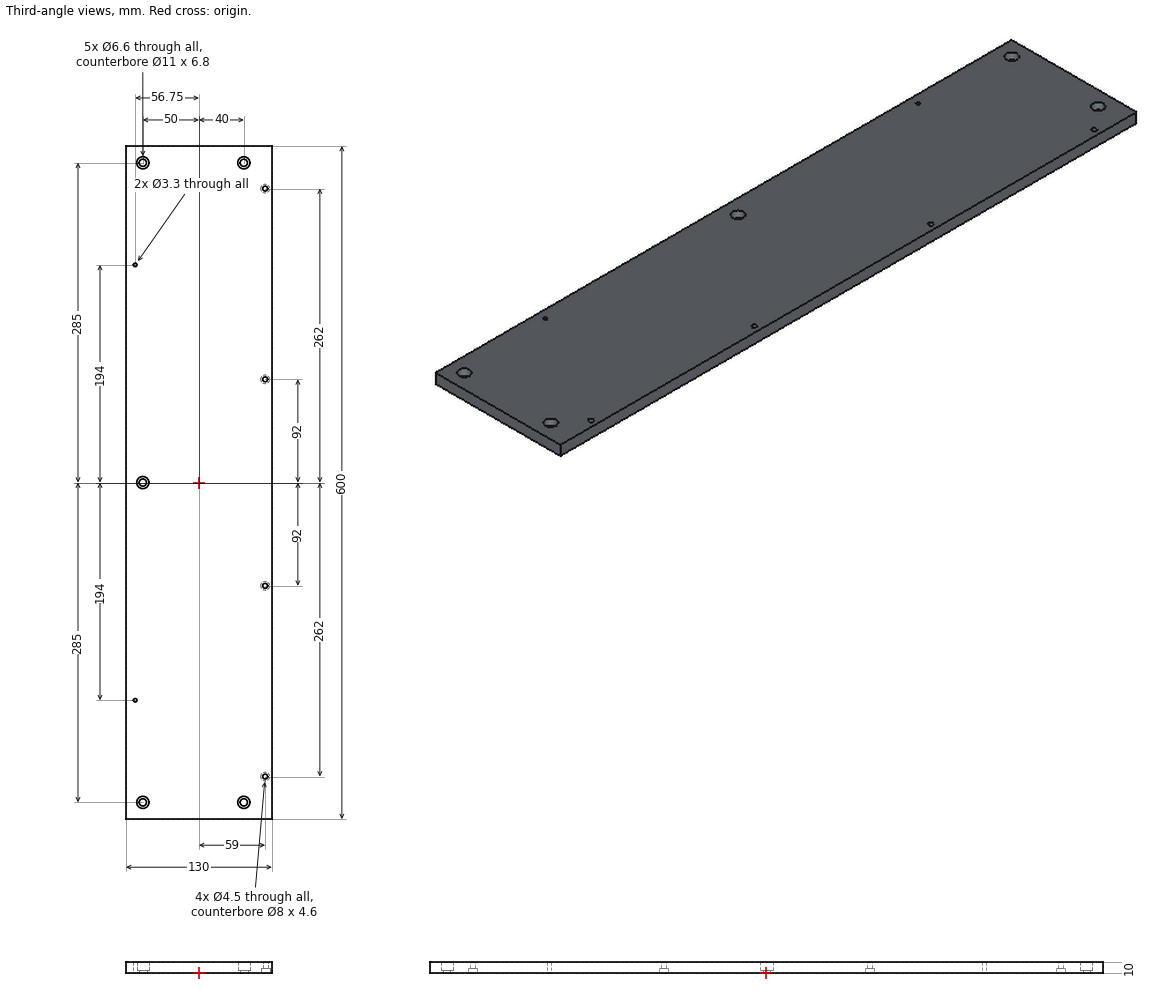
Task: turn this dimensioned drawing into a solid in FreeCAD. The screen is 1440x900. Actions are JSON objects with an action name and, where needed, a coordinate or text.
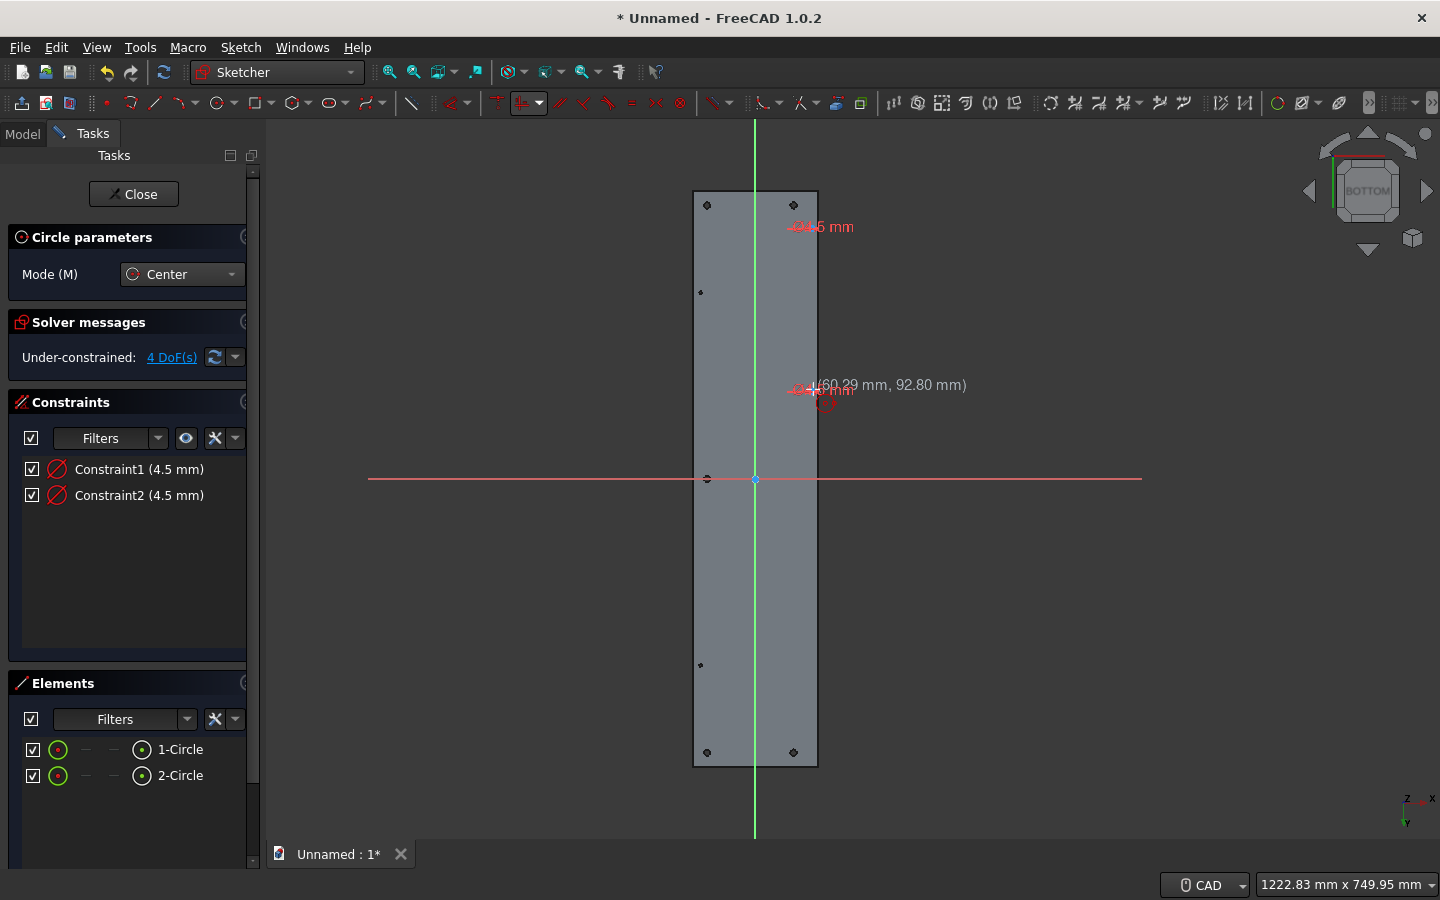
{"action": "scroll", "coordinate": [812, 567], "scroll_direction": "up", "scroll_amount": 12}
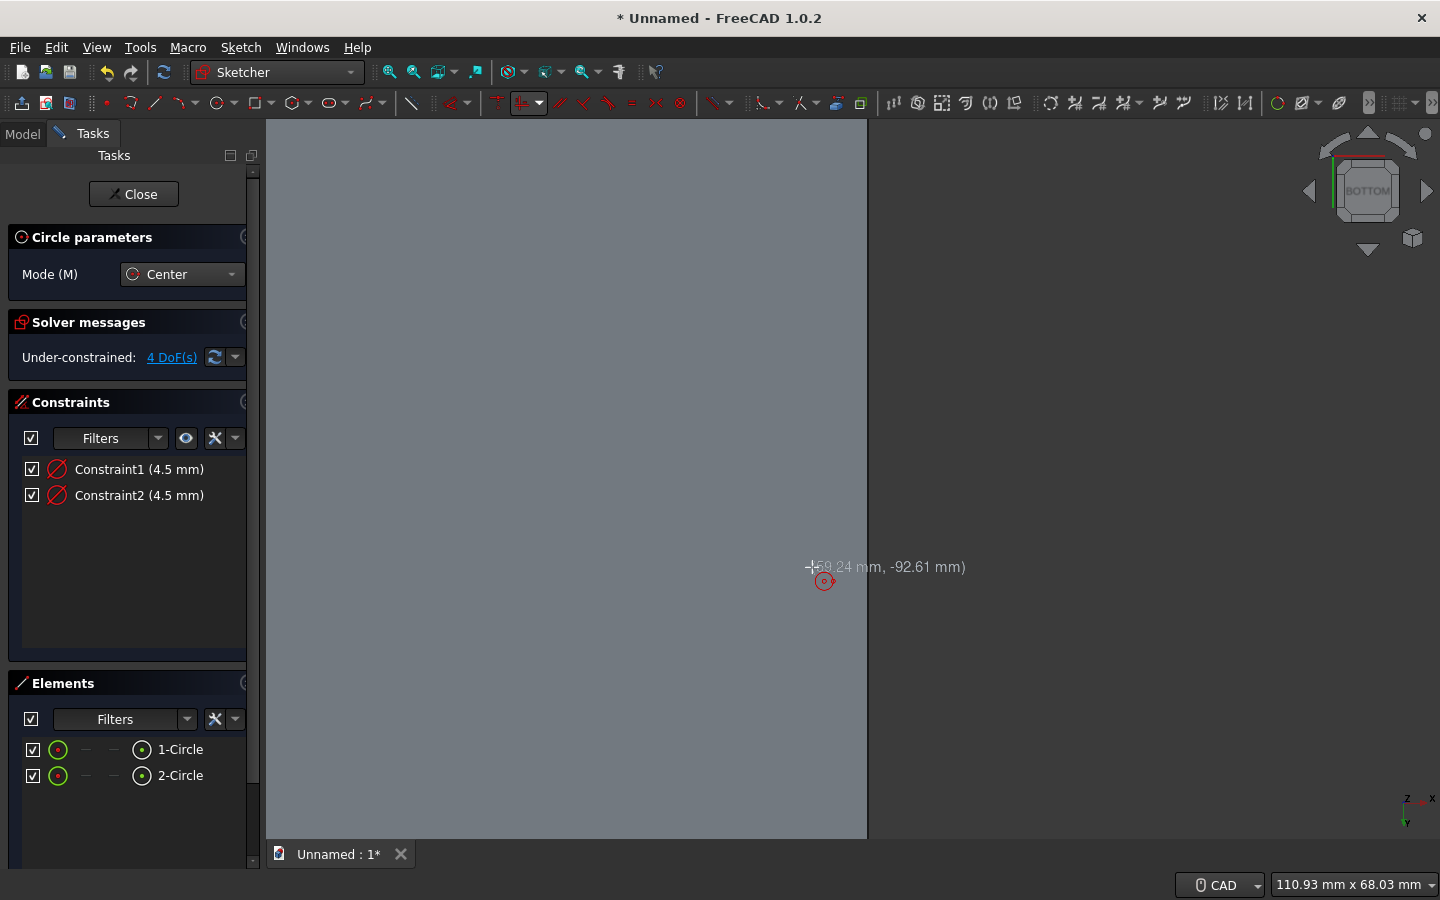
{"action": "scroll", "coordinate": [812, 568], "scroll_direction": "down", "scroll_amount": 12}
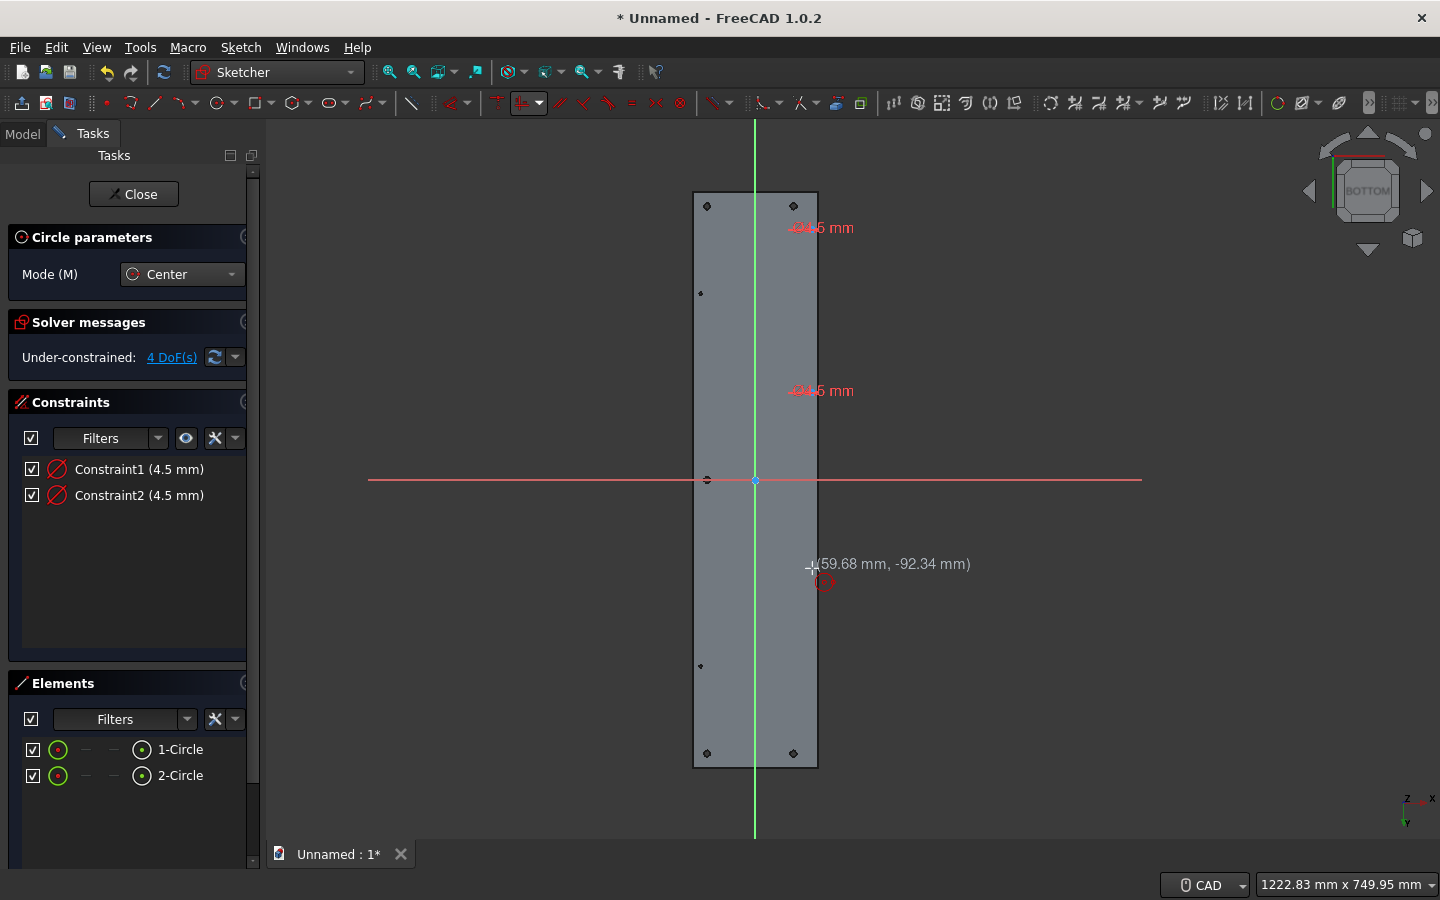
{"action": "left_click", "coordinate": [812, 568]}
{"action": "mouse_move", "coordinate": [813, 567]}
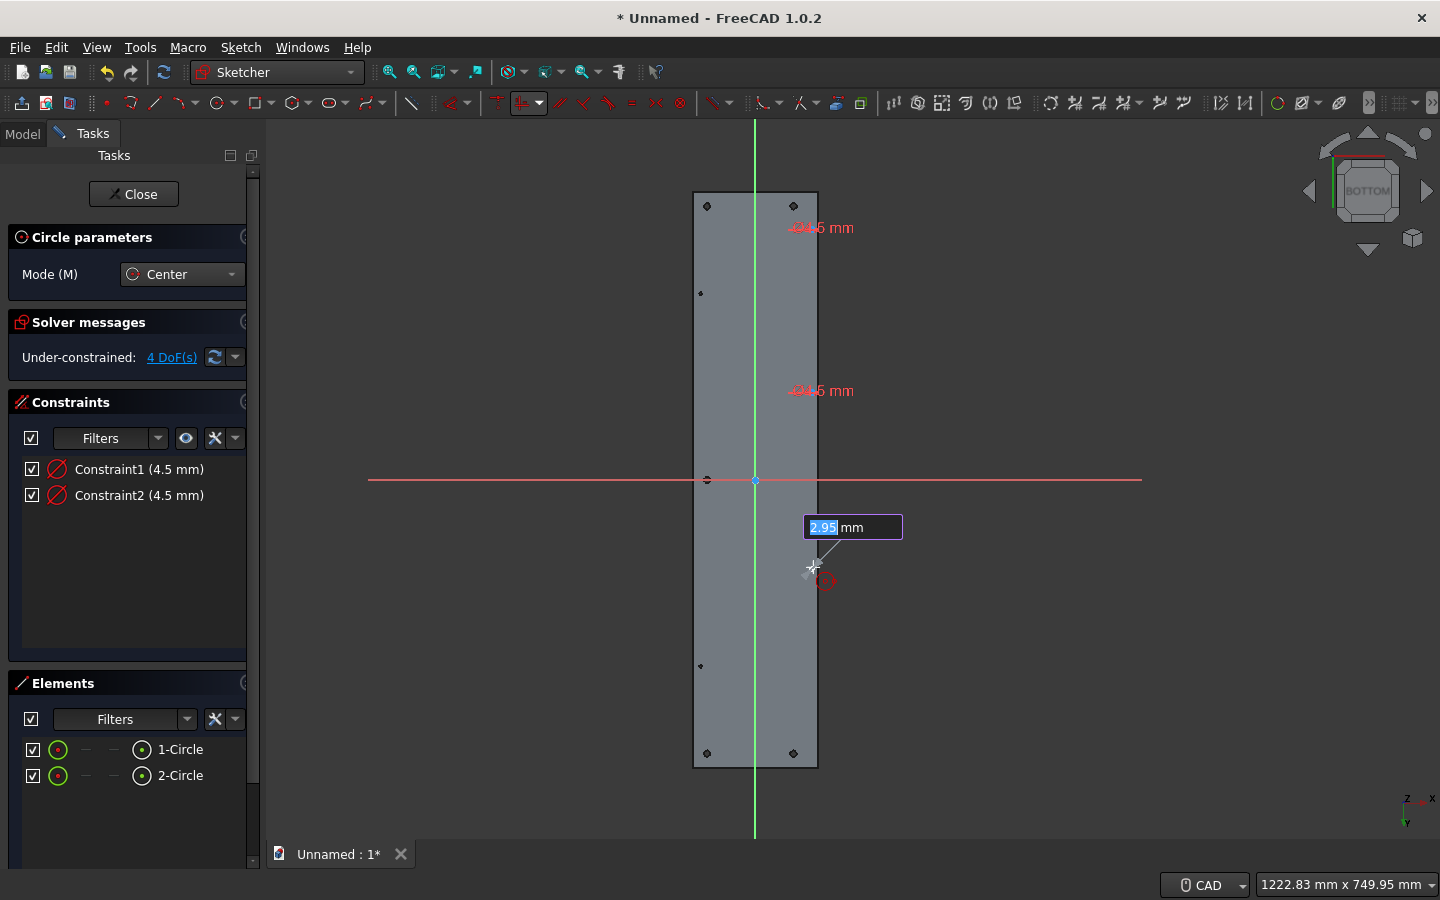
{"action": "type", "text": "4.5"}
{"action": "key", "text": "Return"}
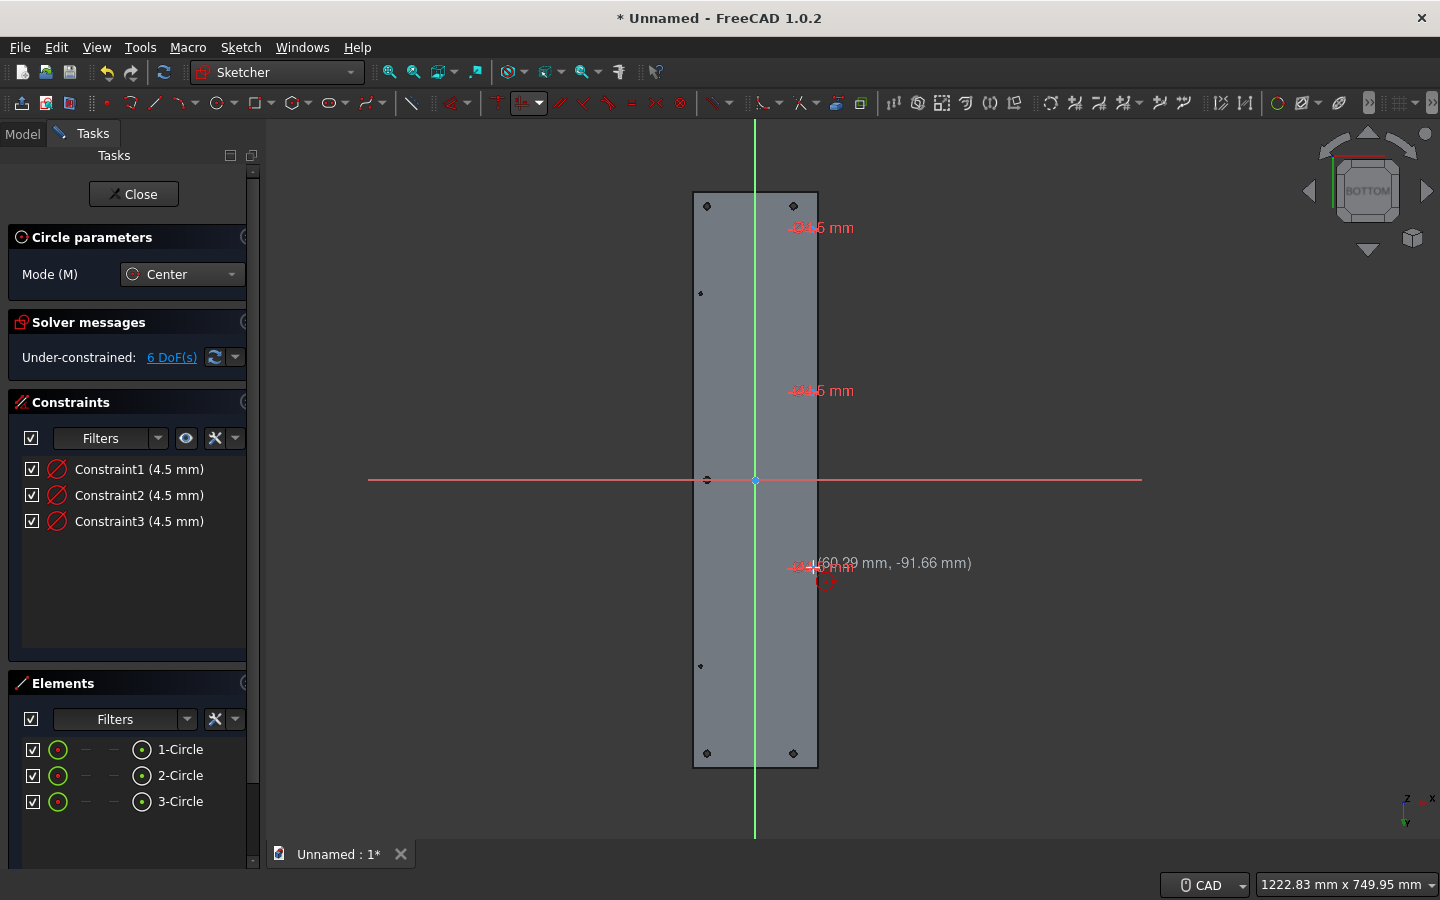
{"action": "scroll", "coordinate": [812, 732], "scroll_direction": "up", "scroll_amount": 12}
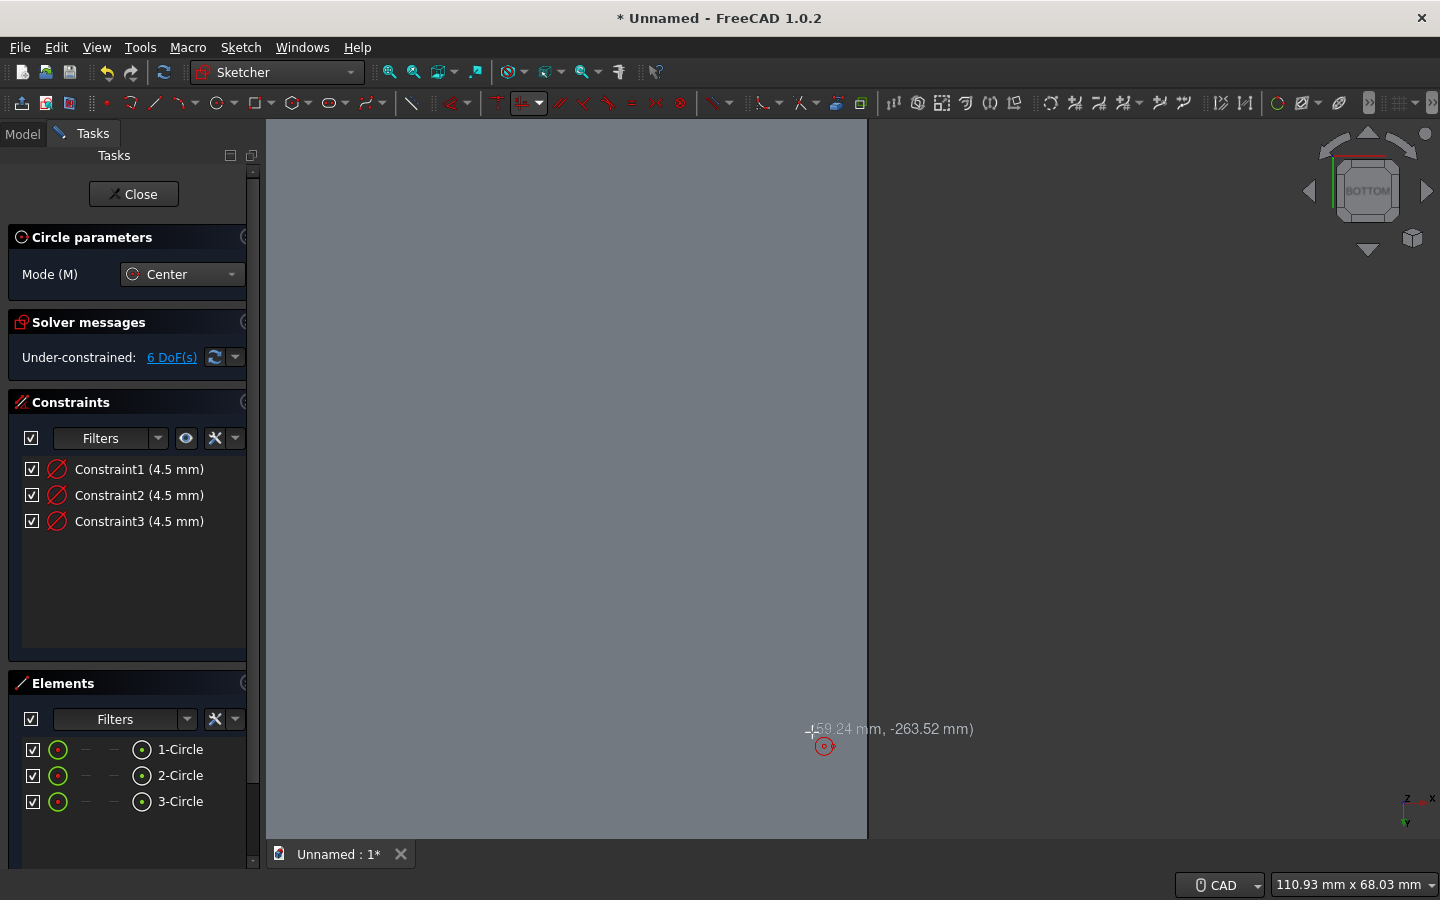
{"action": "scroll", "coordinate": [812, 732], "scroll_direction": "down", "scroll_amount": 12}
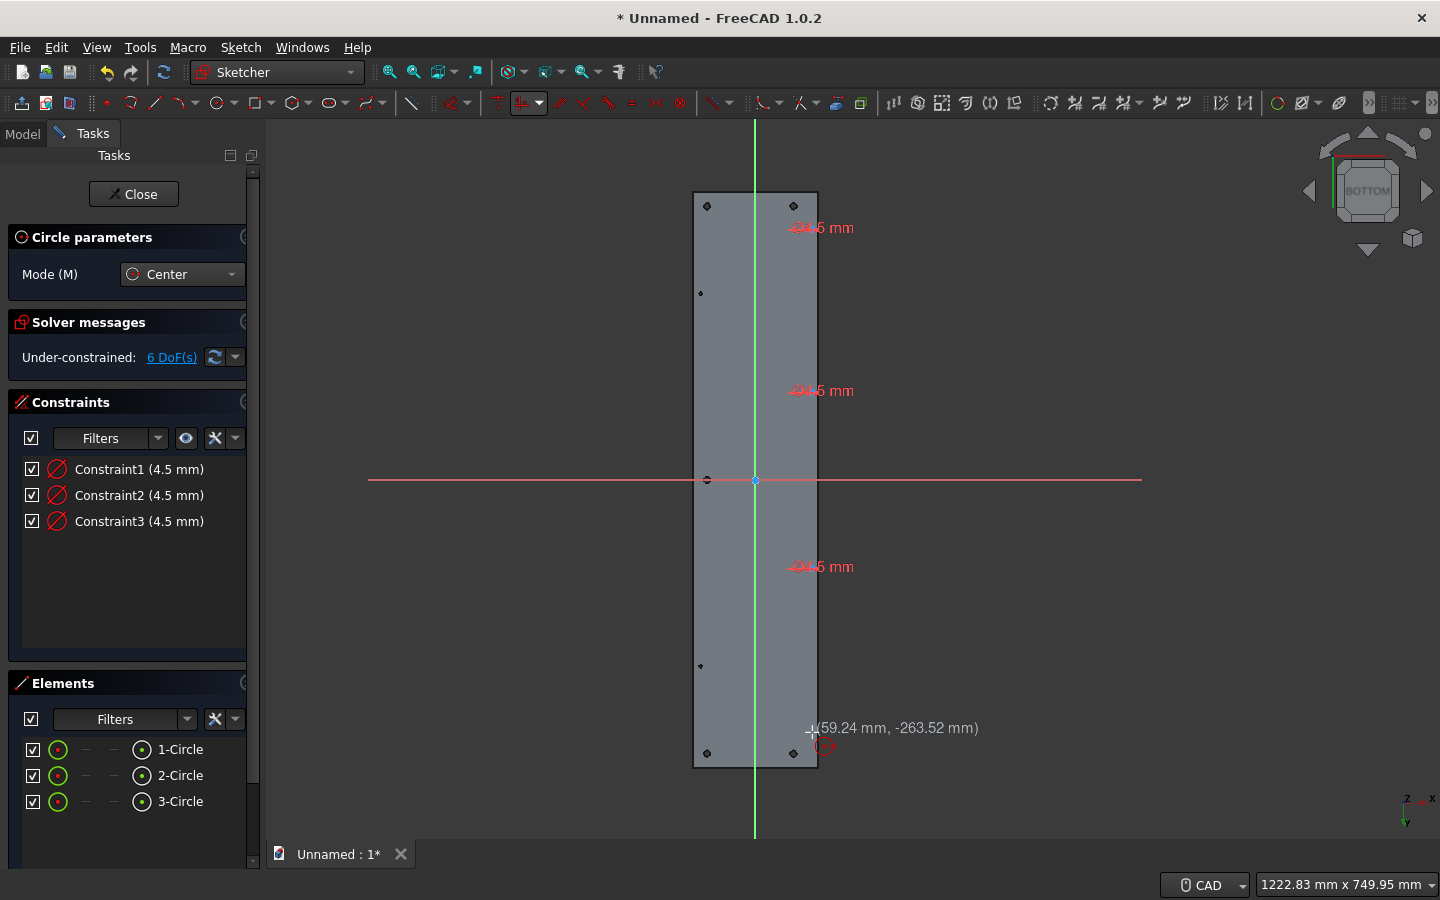
{"action": "left_click", "coordinate": [812, 732]}
{"action": "mouse_move", "coordinate": [813, 730]}